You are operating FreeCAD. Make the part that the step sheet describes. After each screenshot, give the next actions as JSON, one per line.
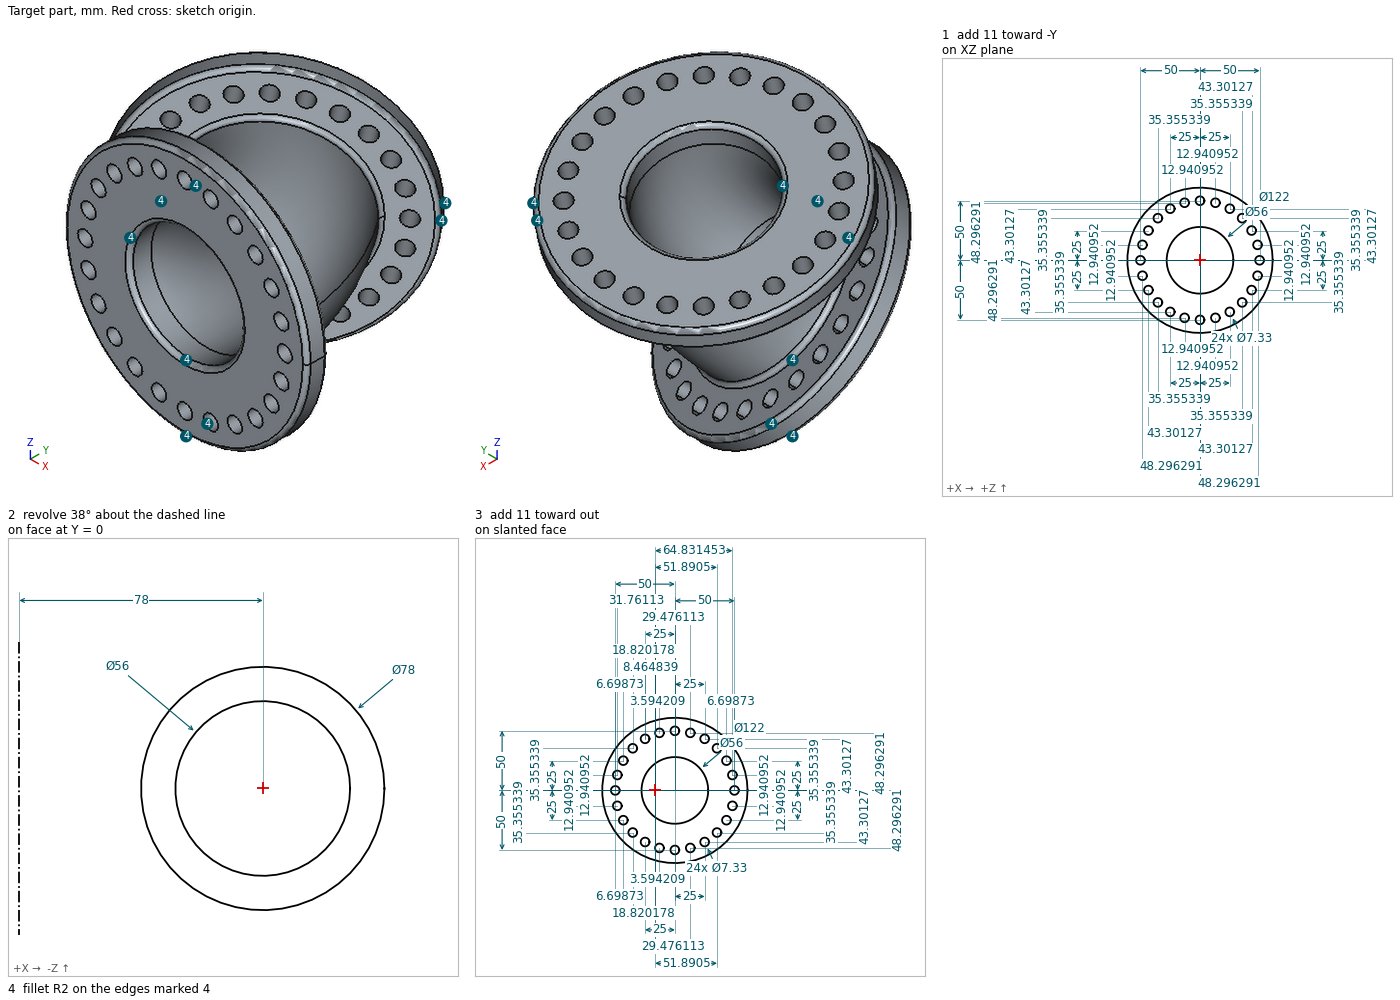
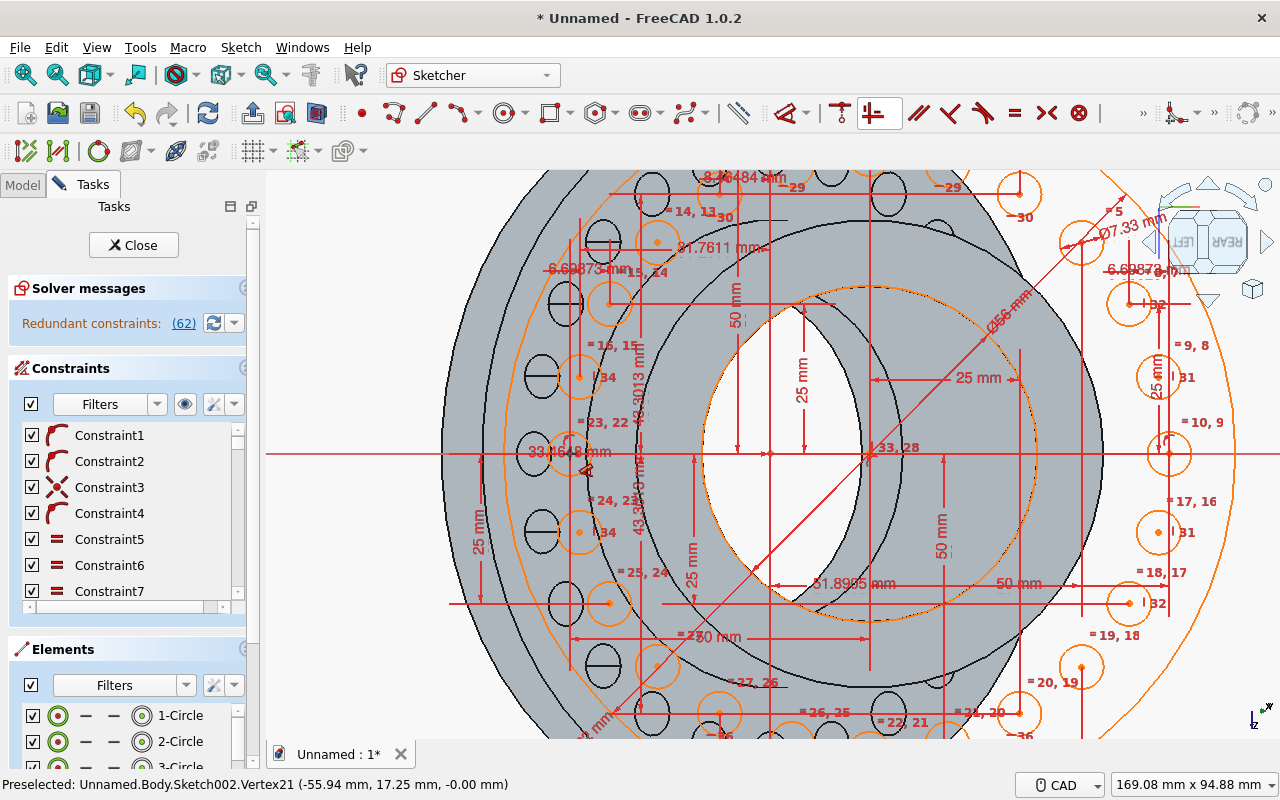
{"action": "left_click", "coordinate": [610, 604]}
{"action": "left_click", "coordinate": [590, 638]}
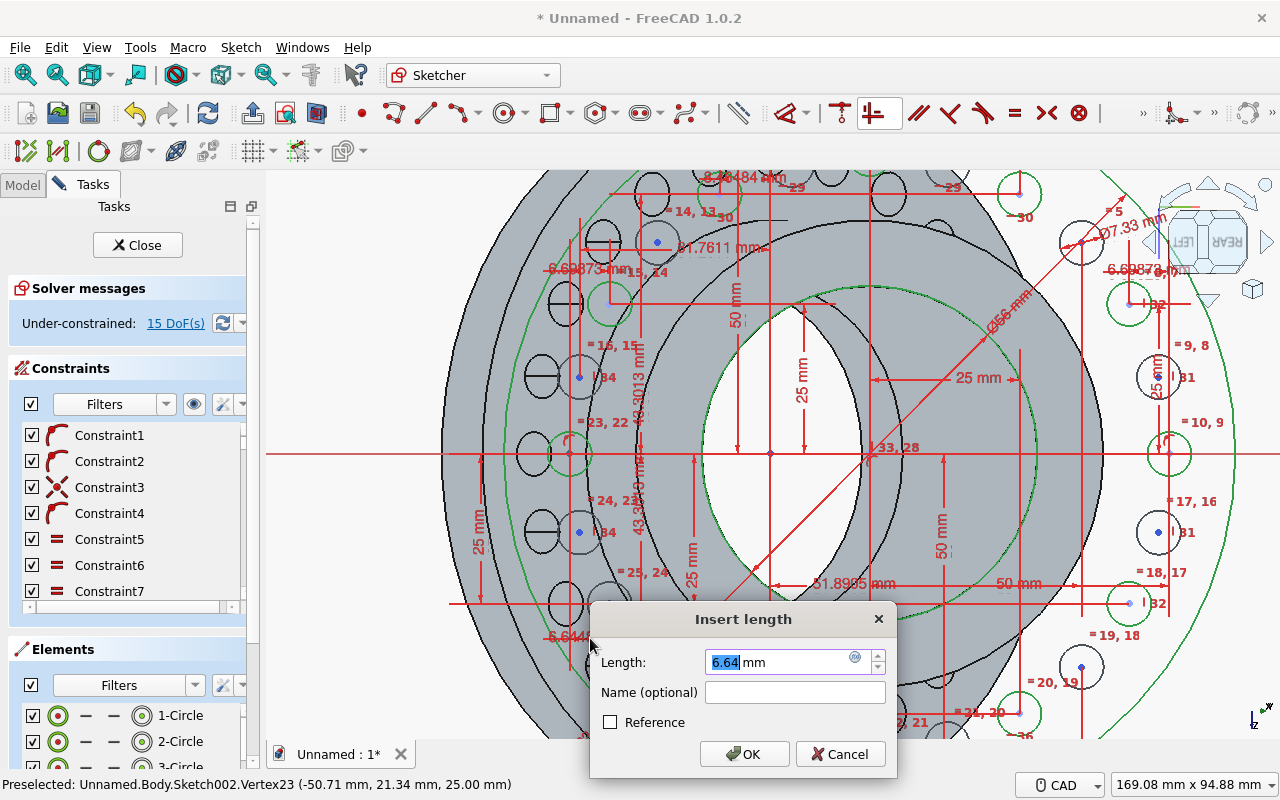
{"action": "type", "text": "6.69873"}
{"action": "key", "text": "Return"}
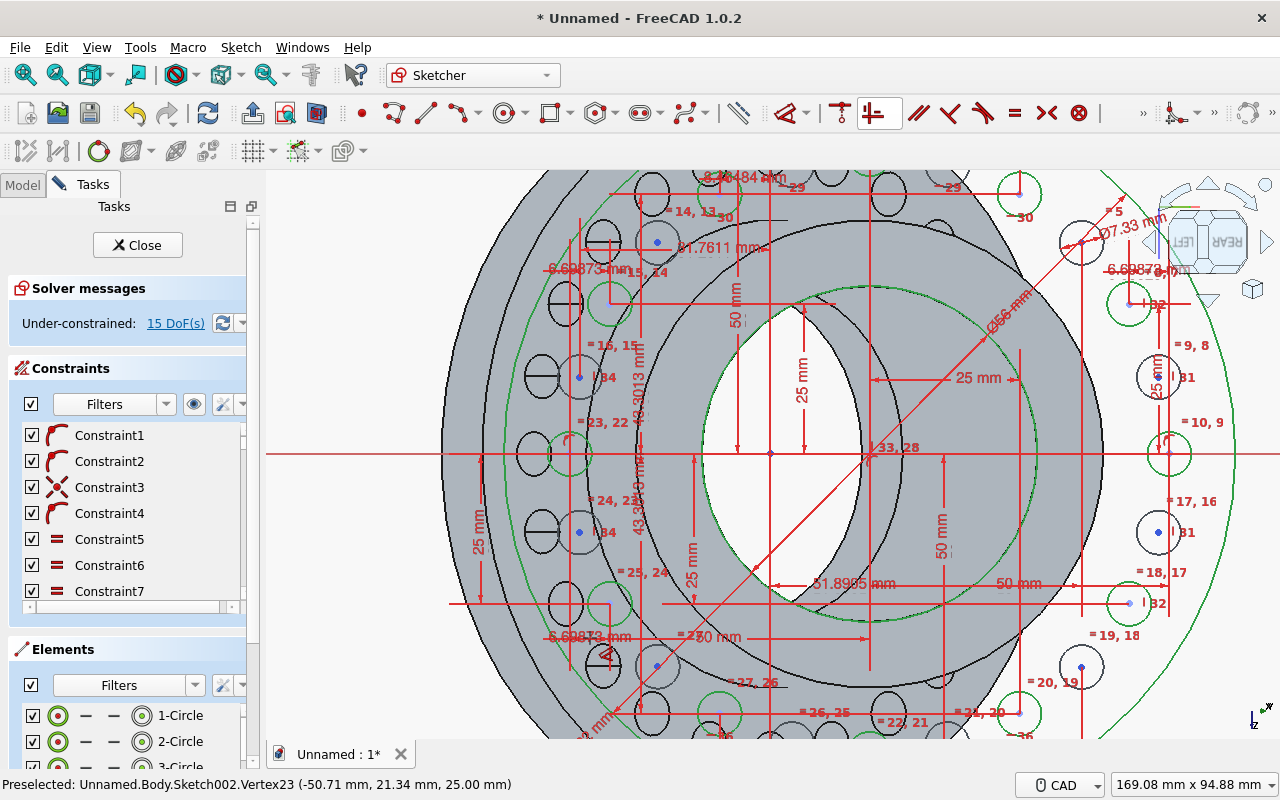
{"action": "left_click", "coordinate": [1082, 243]}
{"action": "left_click", "coordinate": [736, 275]}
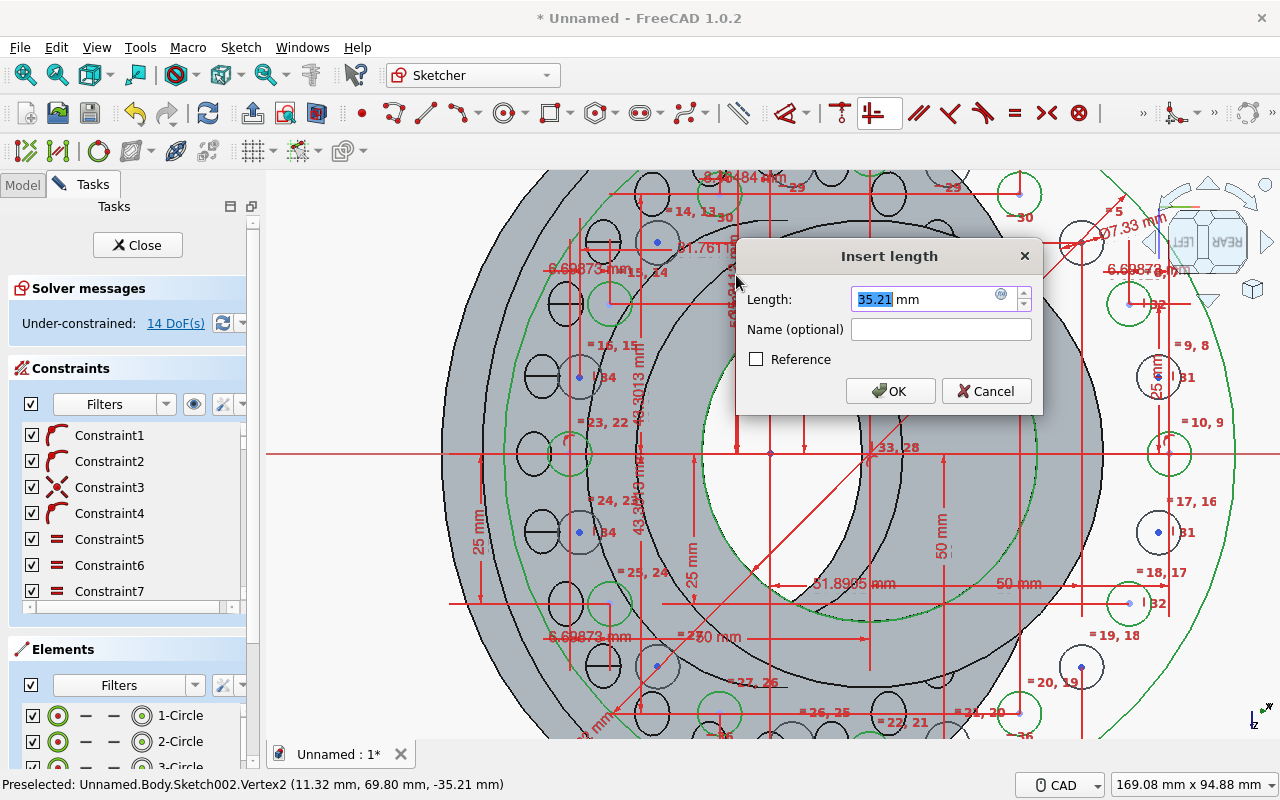
{"action": "type", "text": "35.355339"}
{"action": "key", "text": "Return"}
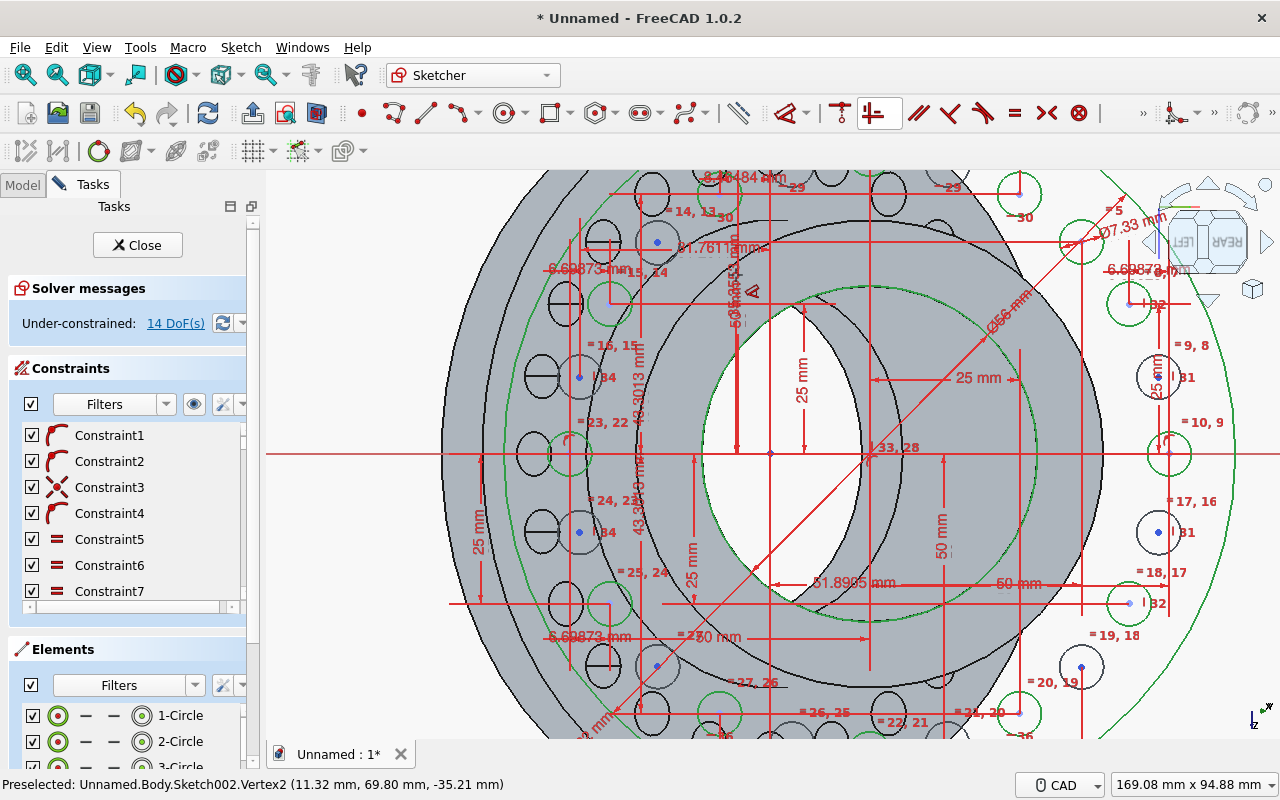
{"action": "scroll", "coordinate": [570, 455], "scroll_direction": "down", "scroll_amount": 4}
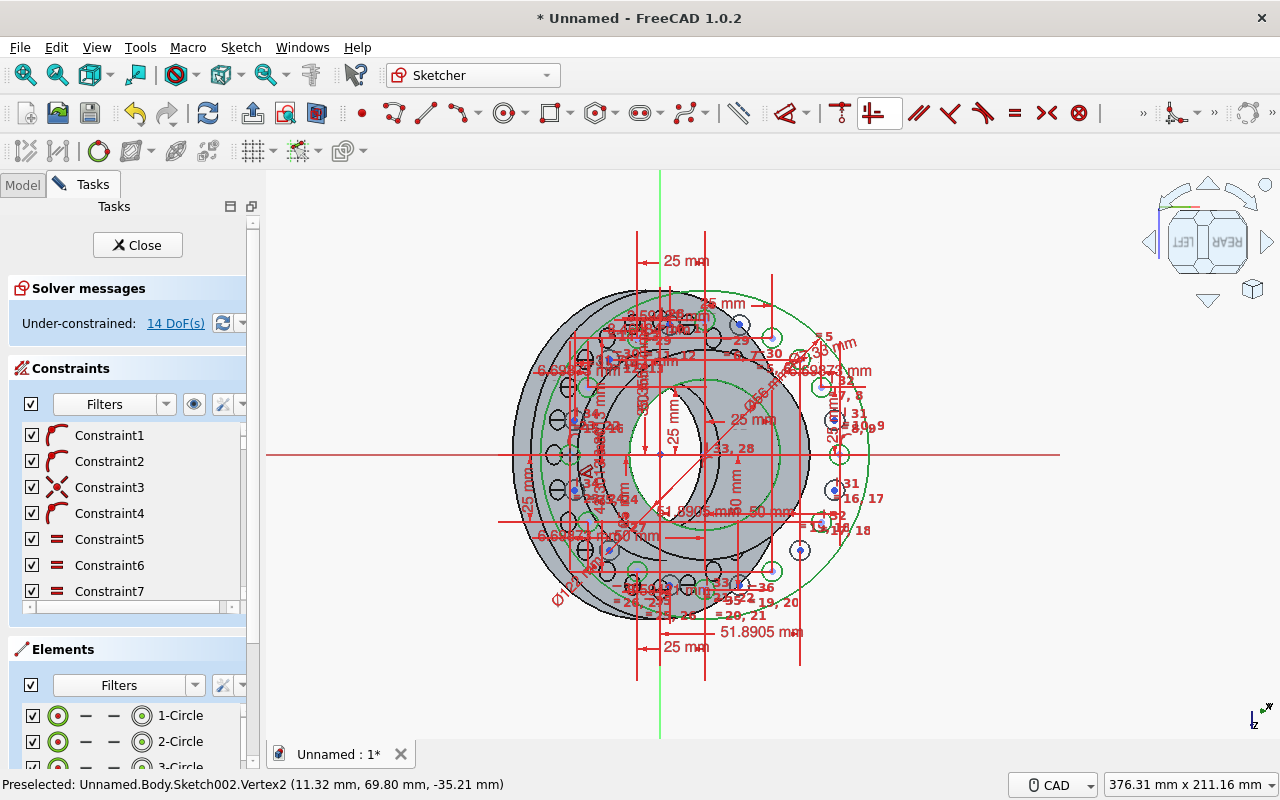
{"action": "left_click", "coordinate": [740, 325]}
{"action": "left_click", "coordinate": [700, 219]}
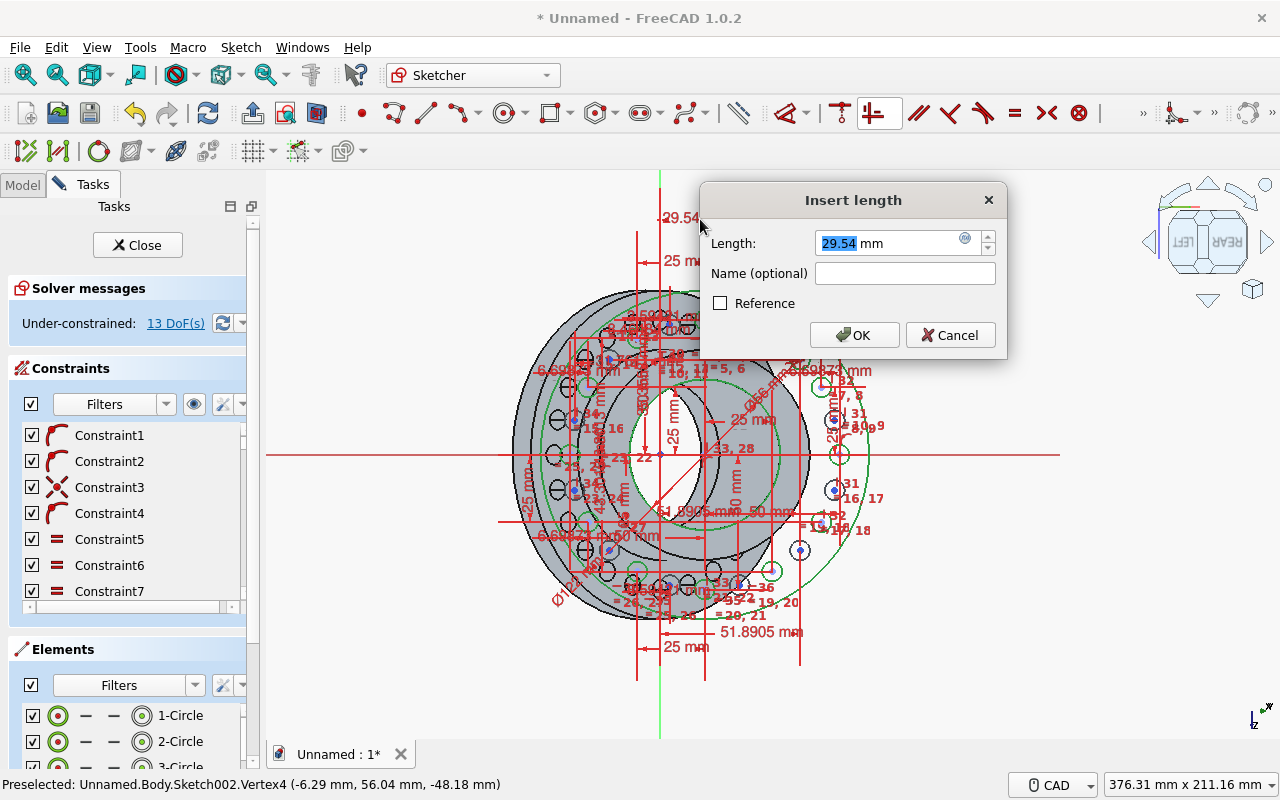
{"action": "type", "text": "29.476113"}
{"action": "key", "text": "Return"}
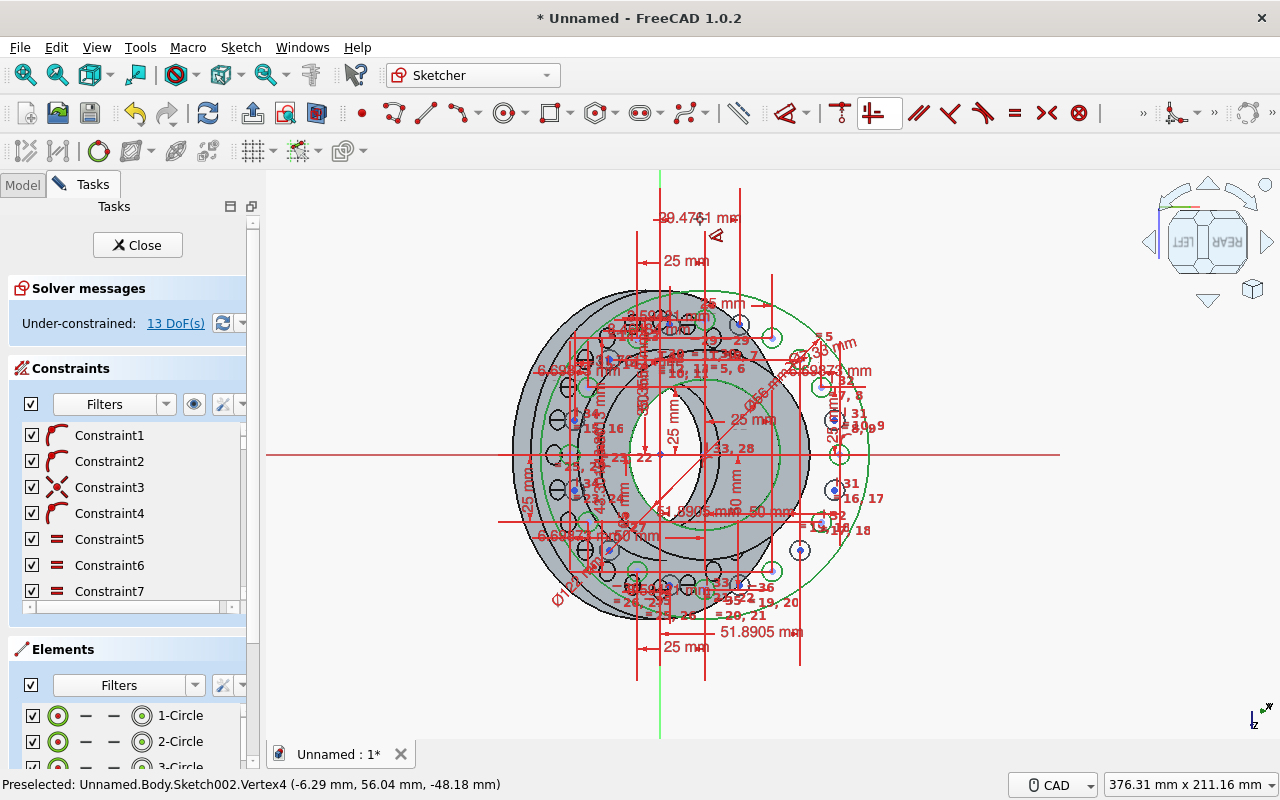
{"action": "left_click", "coordinate": [740, 325]}
{"action": "left_click", "coordinate": [554, 344]}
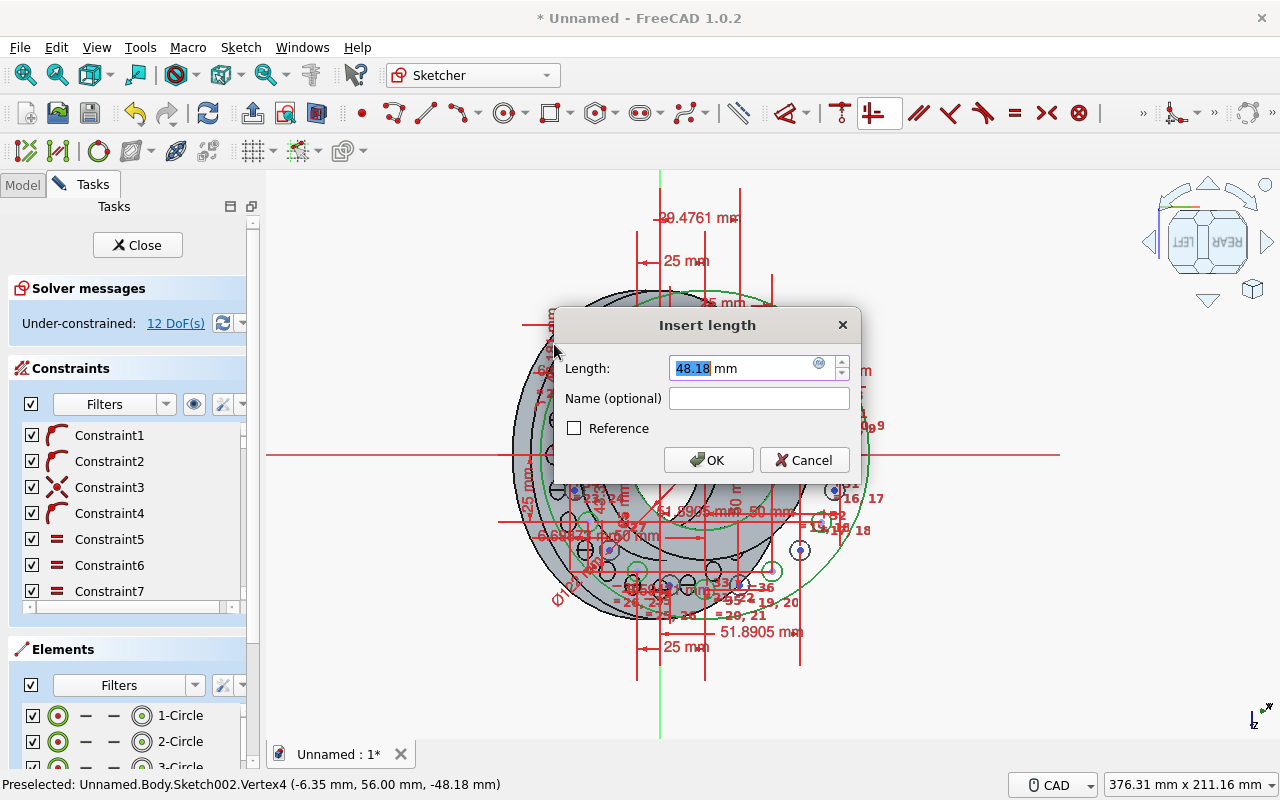
{"action": "type", "text": "48.296291"}
{"action": "key", "text": "Return"}